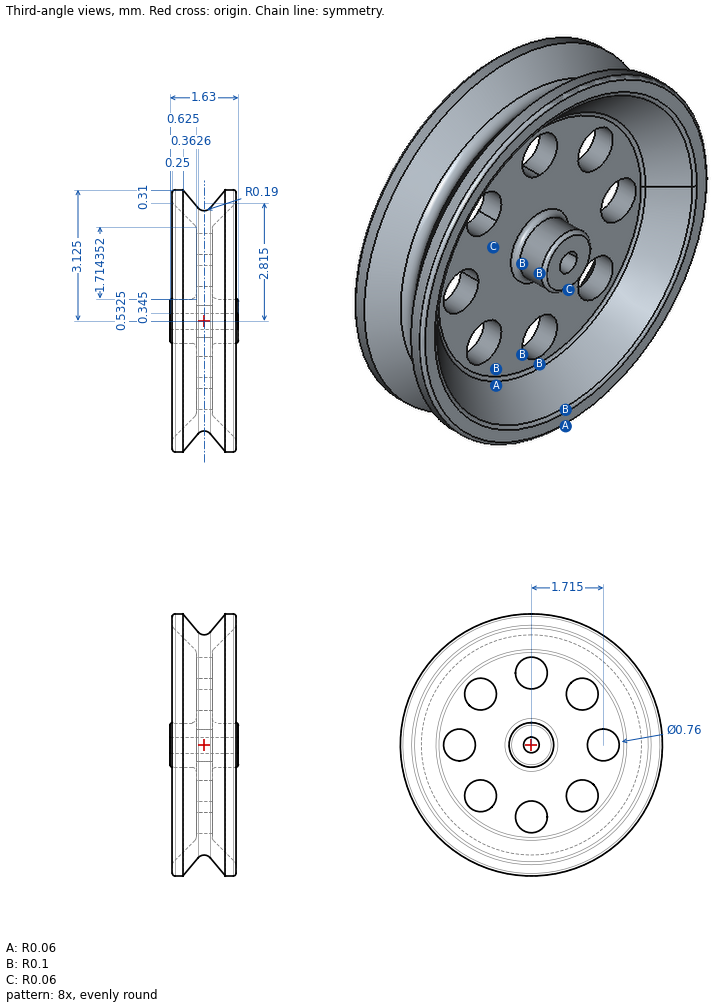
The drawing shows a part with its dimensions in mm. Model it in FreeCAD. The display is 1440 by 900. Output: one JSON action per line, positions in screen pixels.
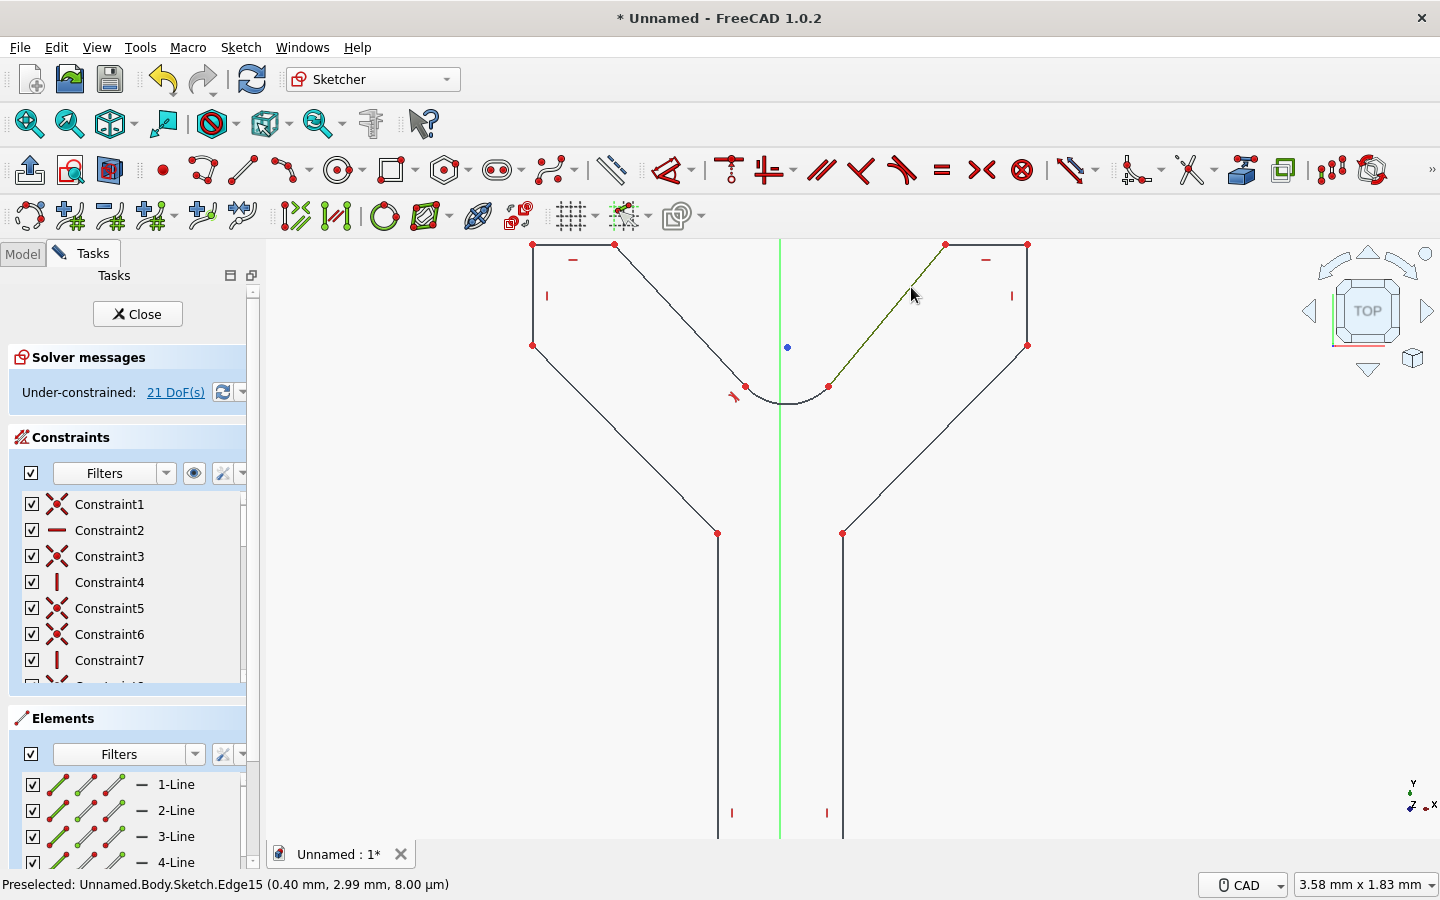
{"action": "left_click", "coordinate": [769, 401]}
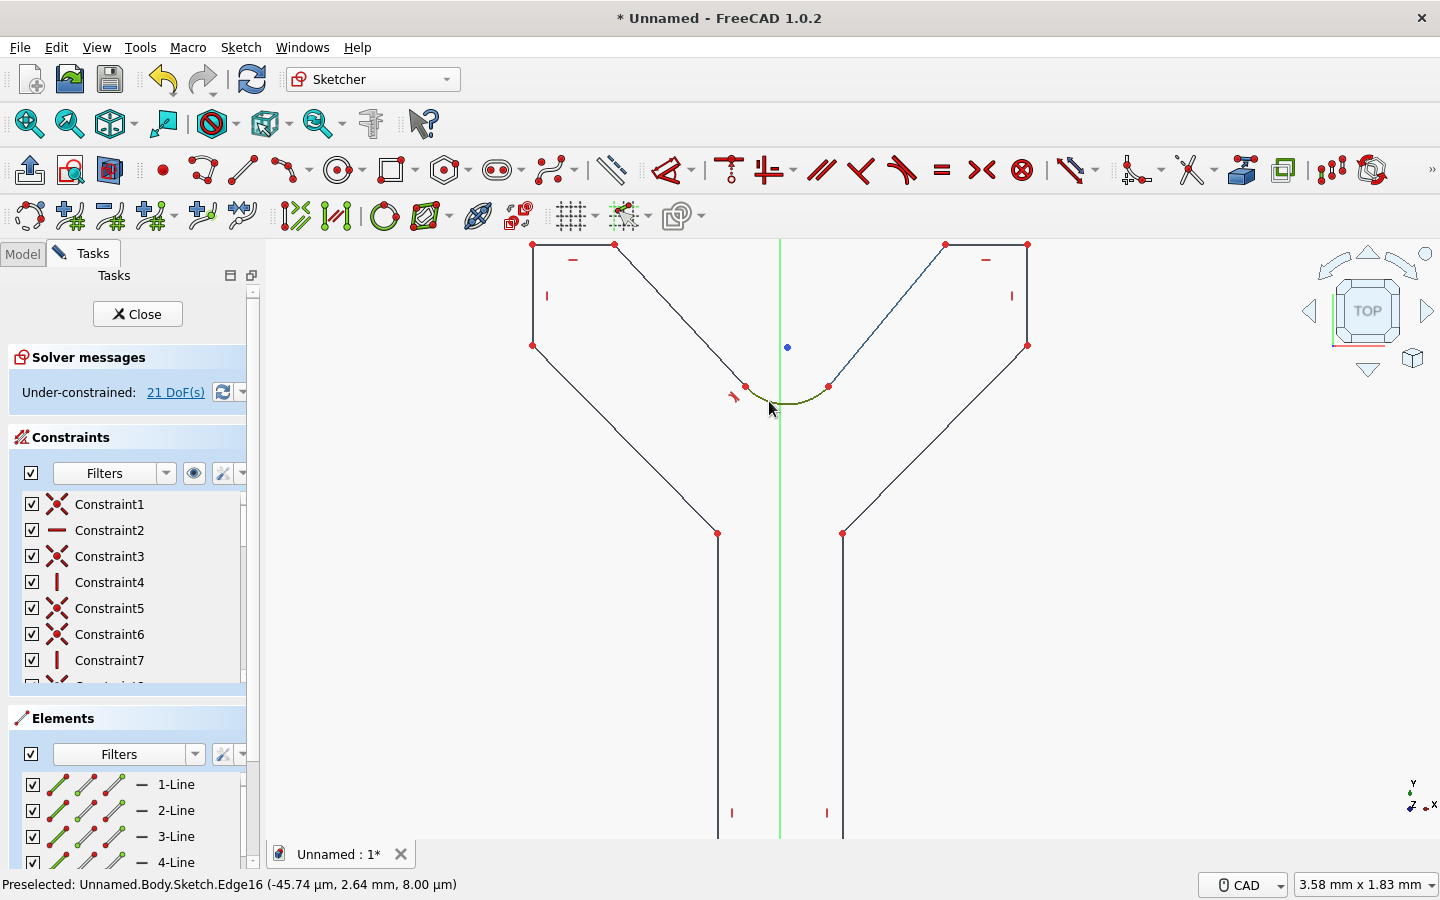
{"action": "key", "text": "t"}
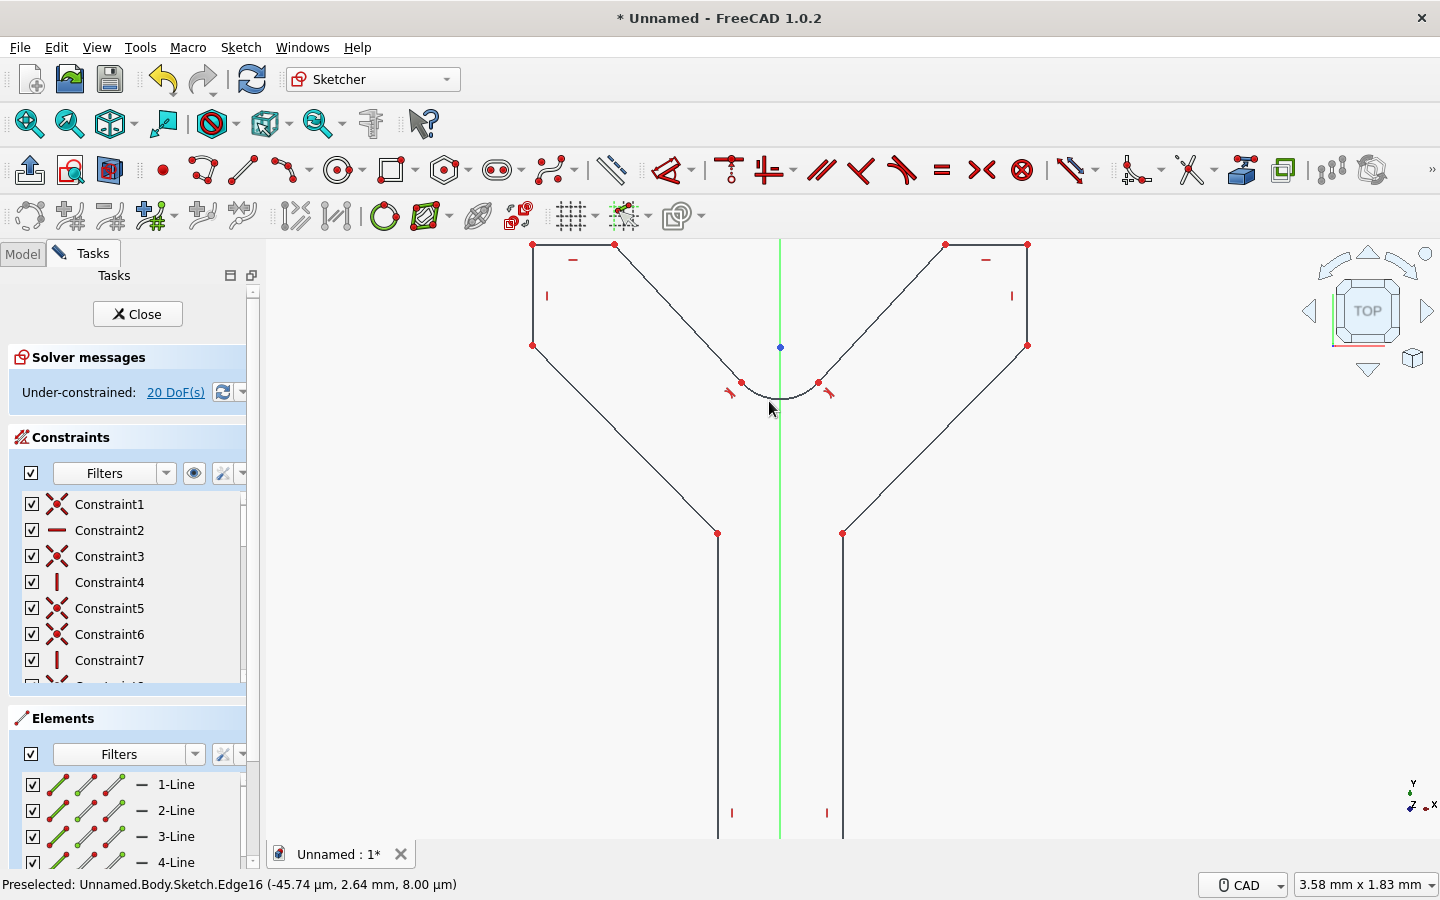
{"action": "left_click", "coordinate": [780, 347]}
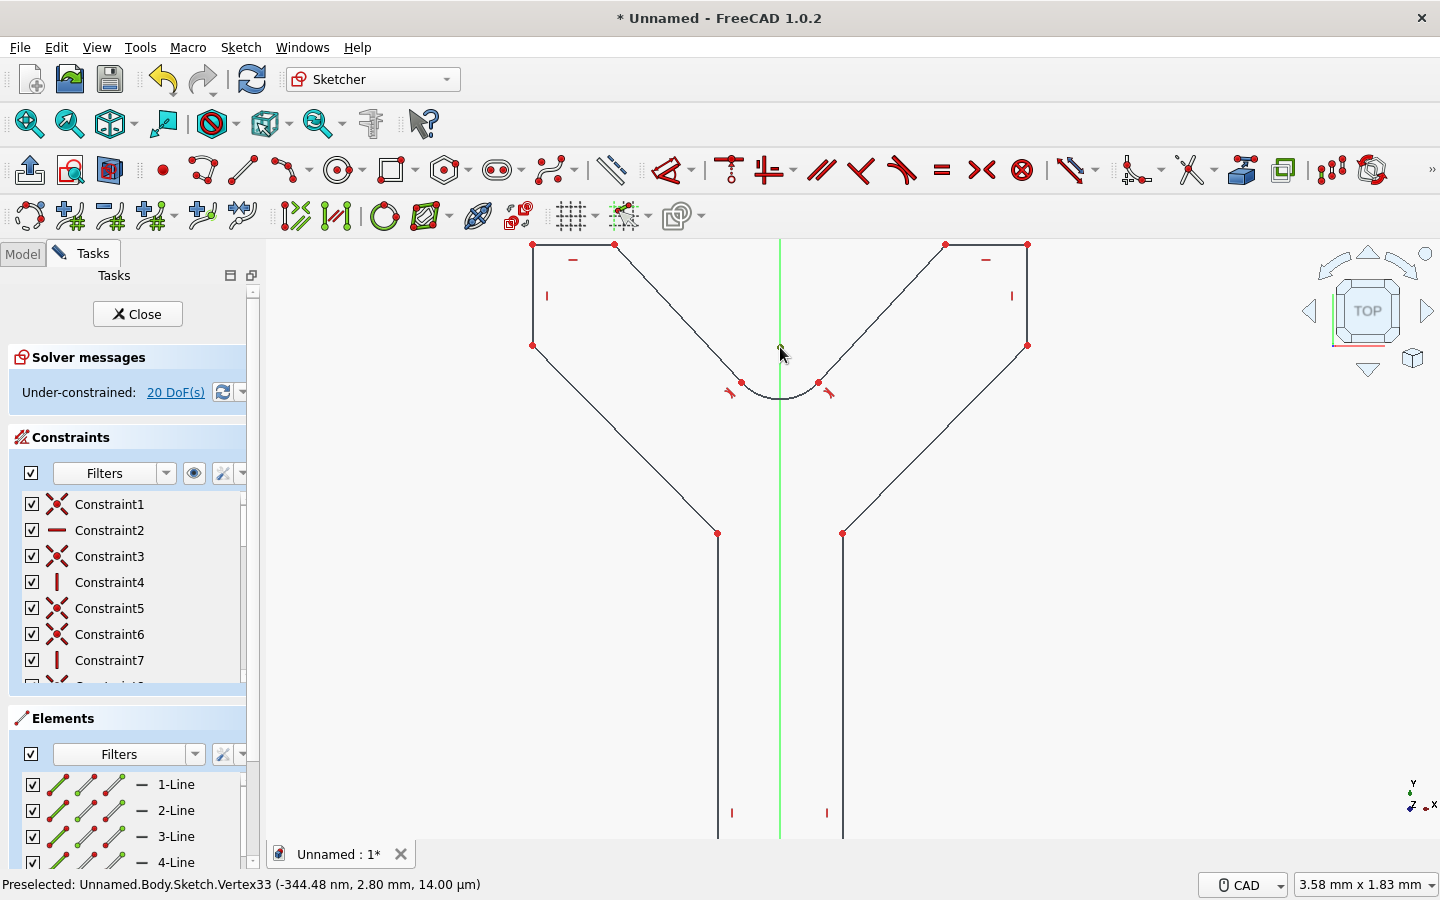
{"action": "left_click", "coordinate": [780, 772]}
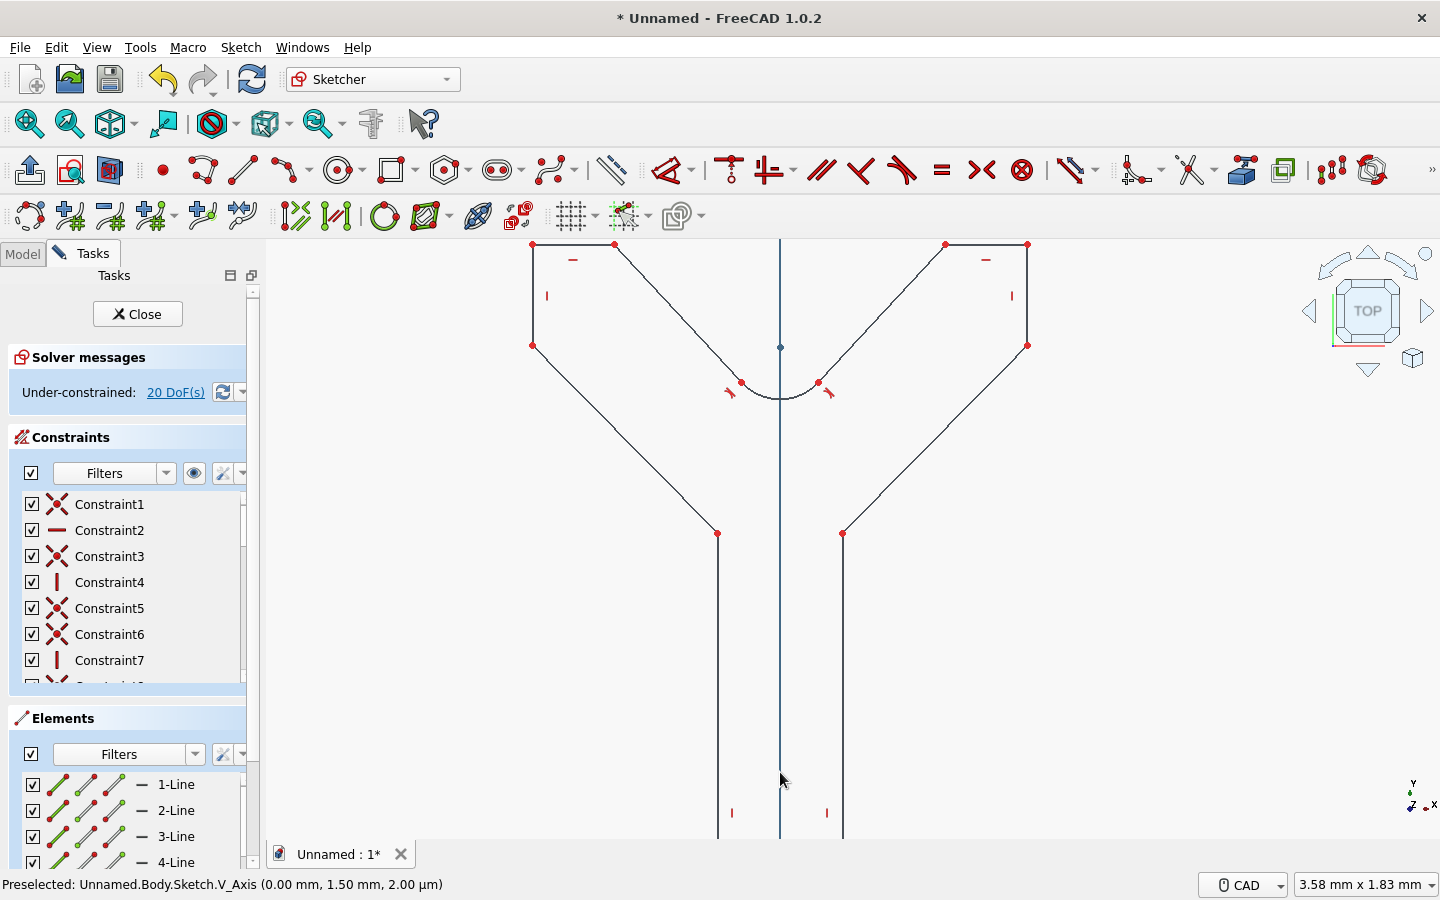
{"action": "left_click", "coordinate": [730, 170]}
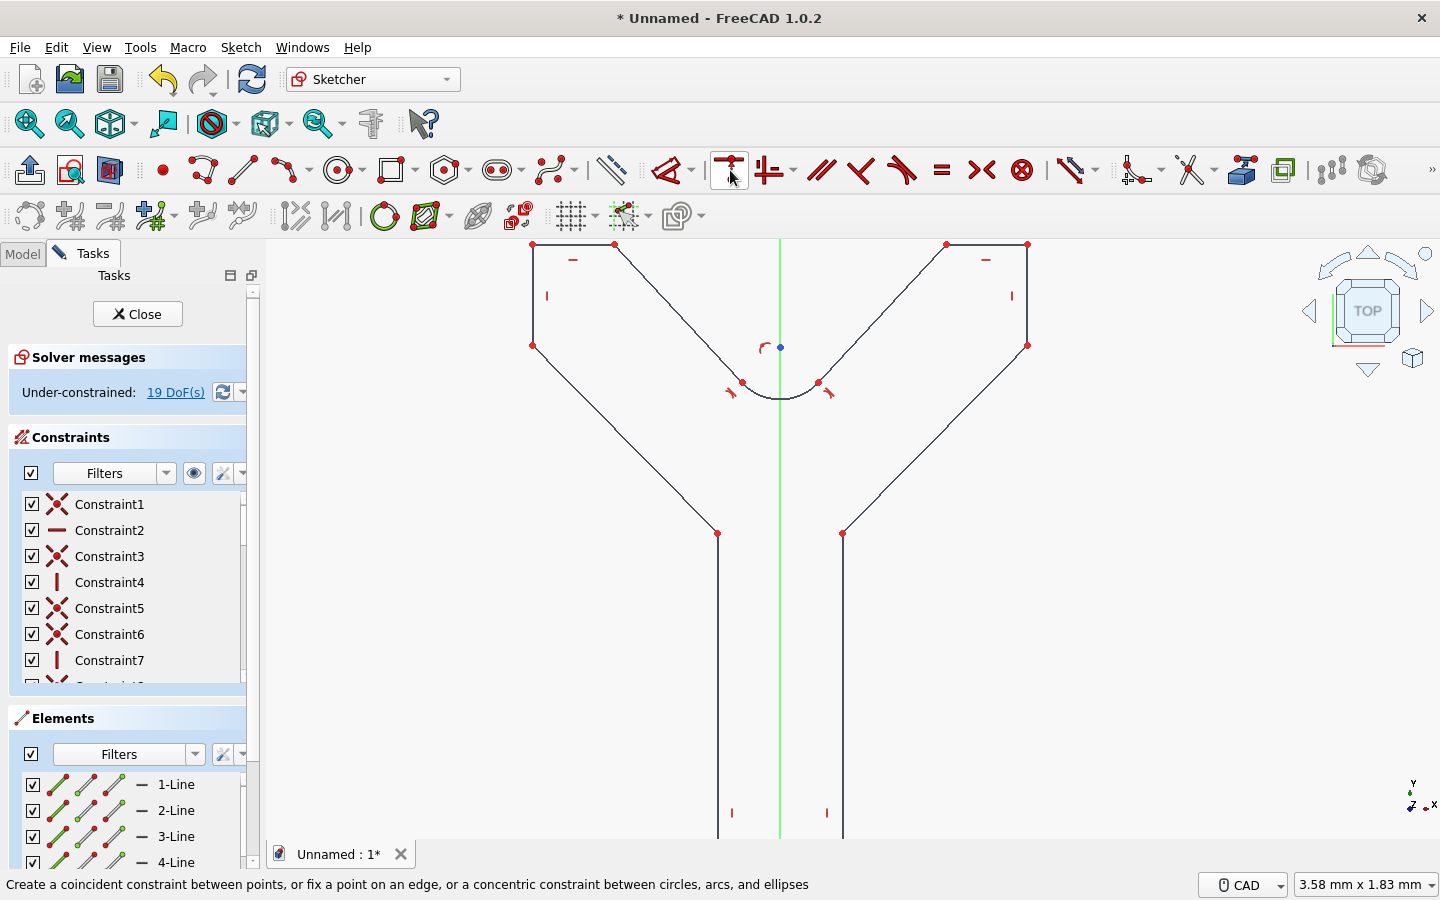
{"action": "scroll", "coordinate": [787, 414], "scroll_direction": "down", "scroll_amount": 5}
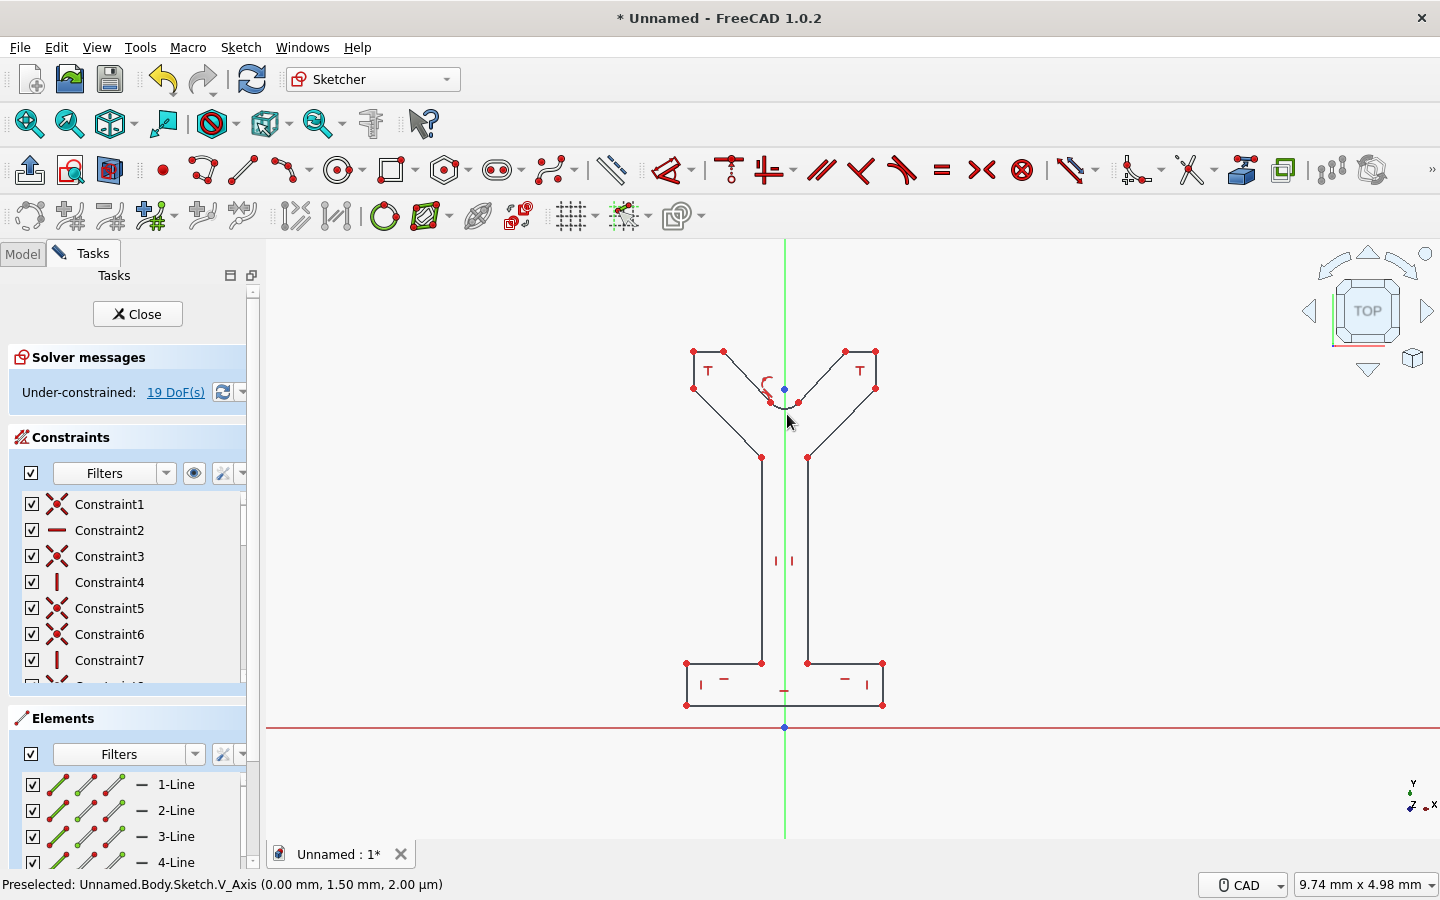
{"action": "left_click", "coordinate": [687, 664]}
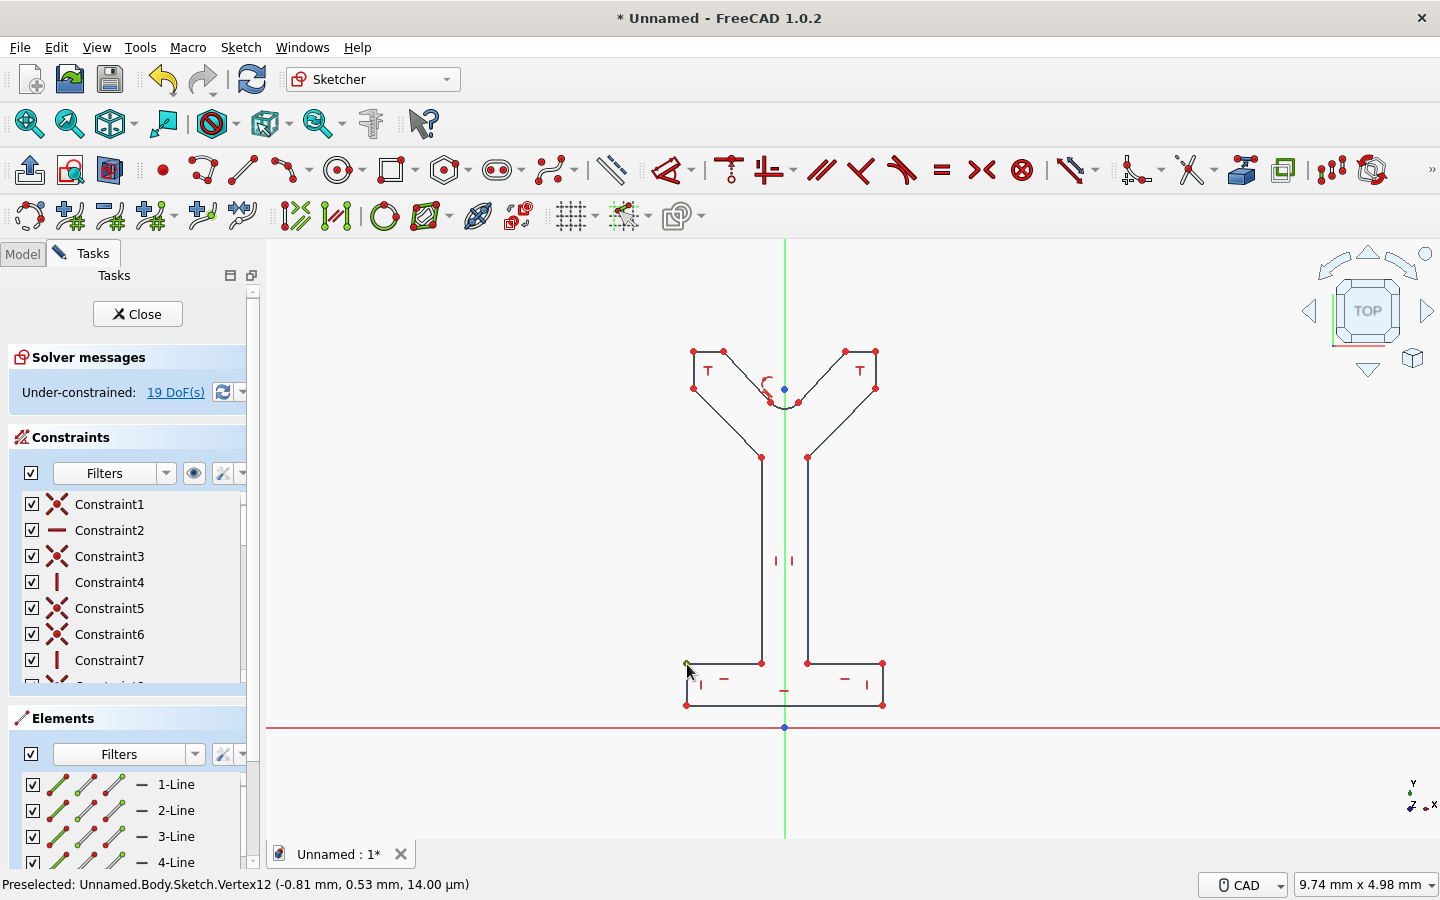
{"action": "left_click", "coordinate": [883, 664]}